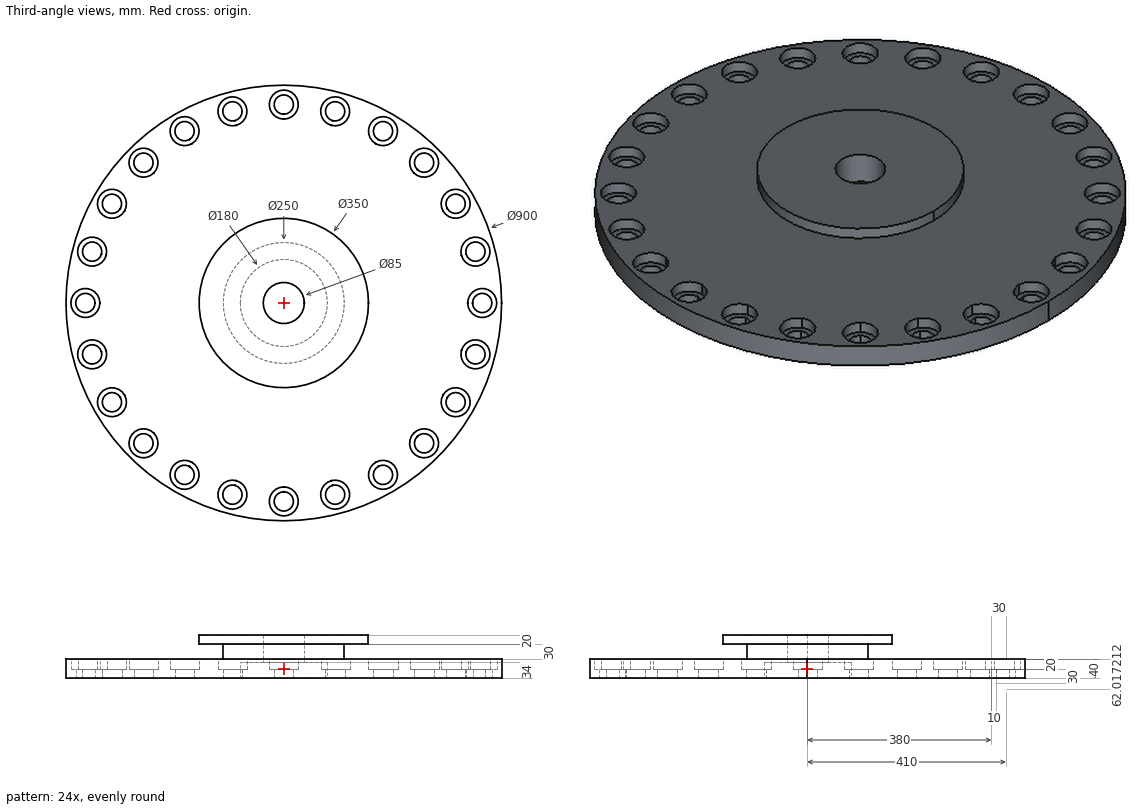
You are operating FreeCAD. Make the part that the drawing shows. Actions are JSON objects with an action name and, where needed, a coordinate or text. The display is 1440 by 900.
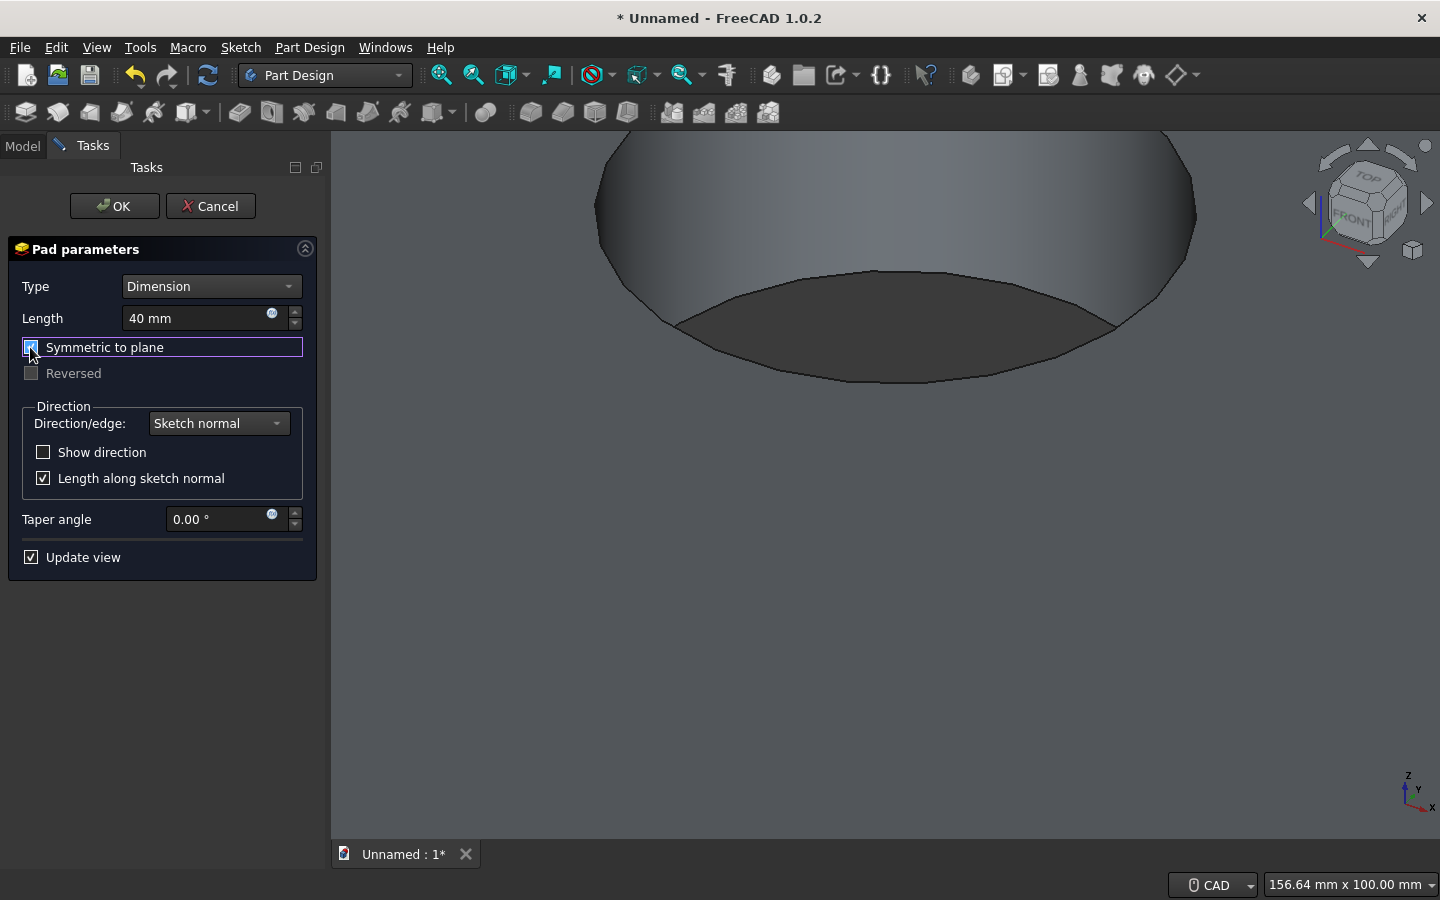
{"action": "left_click", "coordinate": [115, 206]}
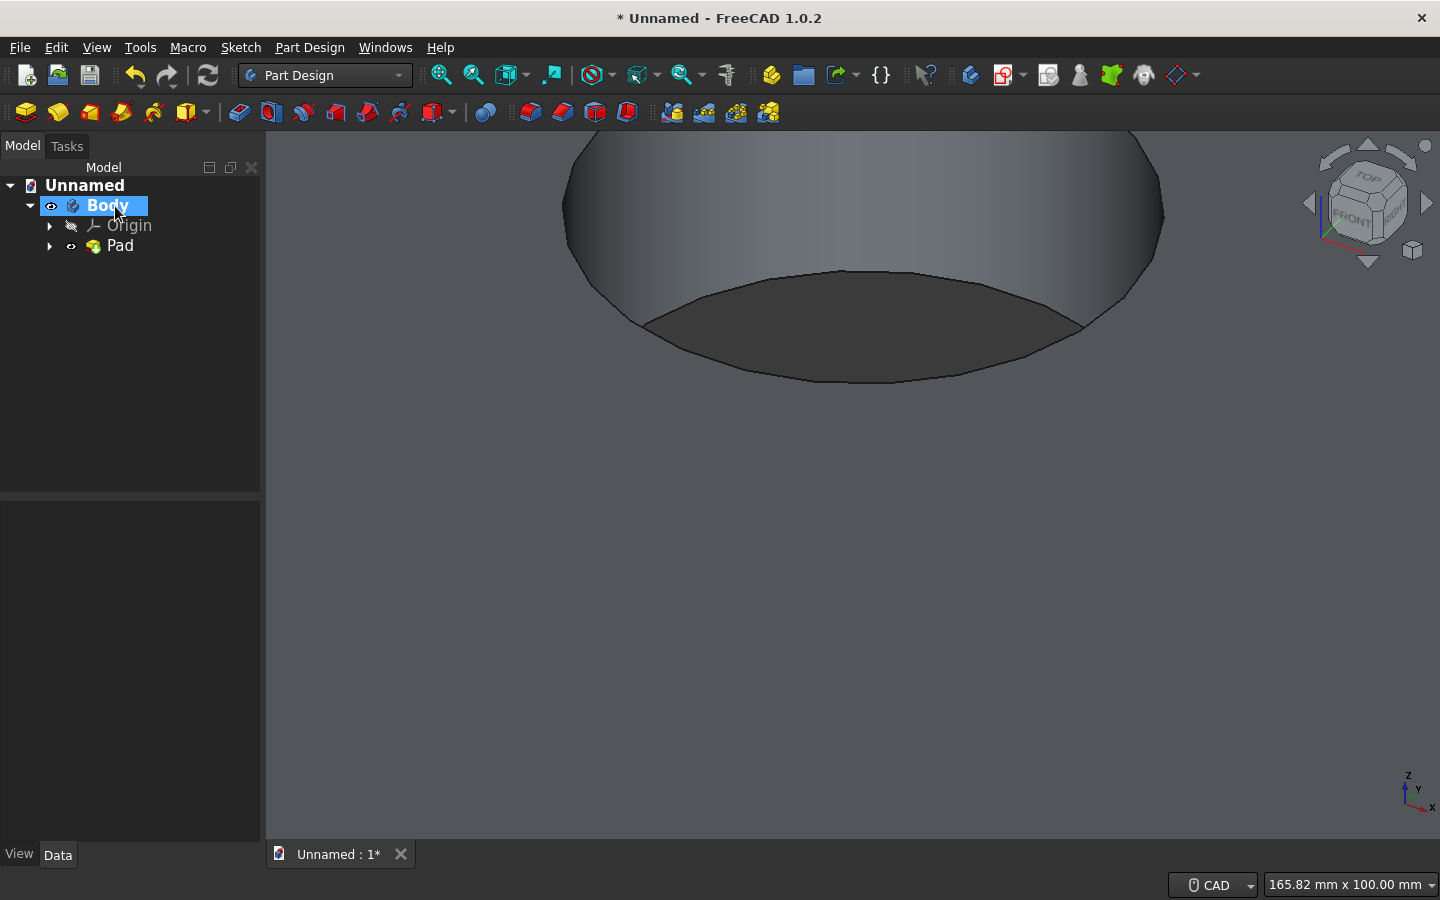
{"action": "key", "text": "v f"}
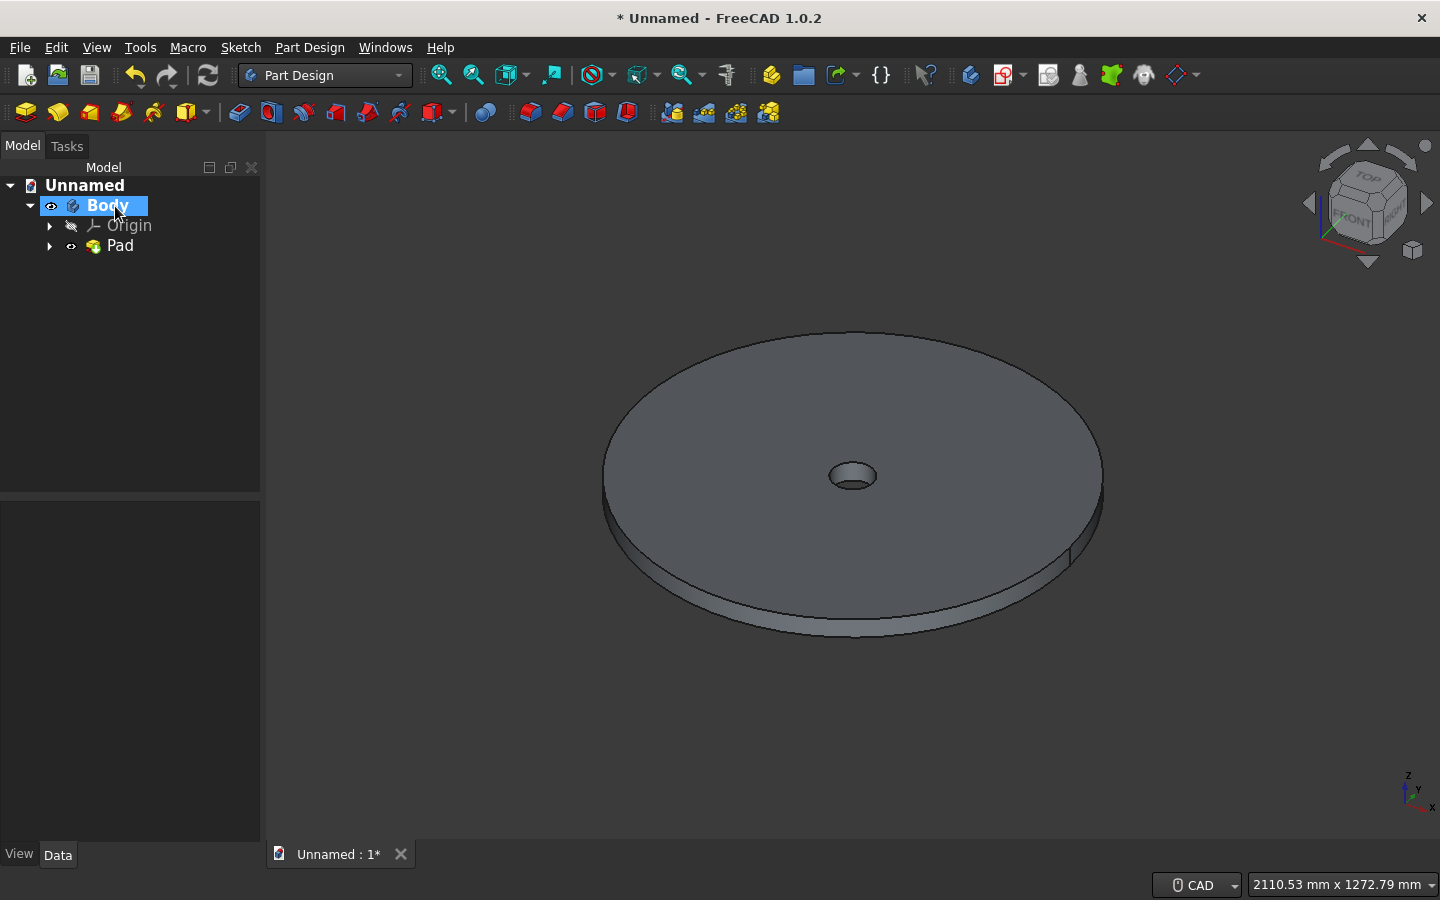
{"action": "left_click", "coordinate": [1004, 76]}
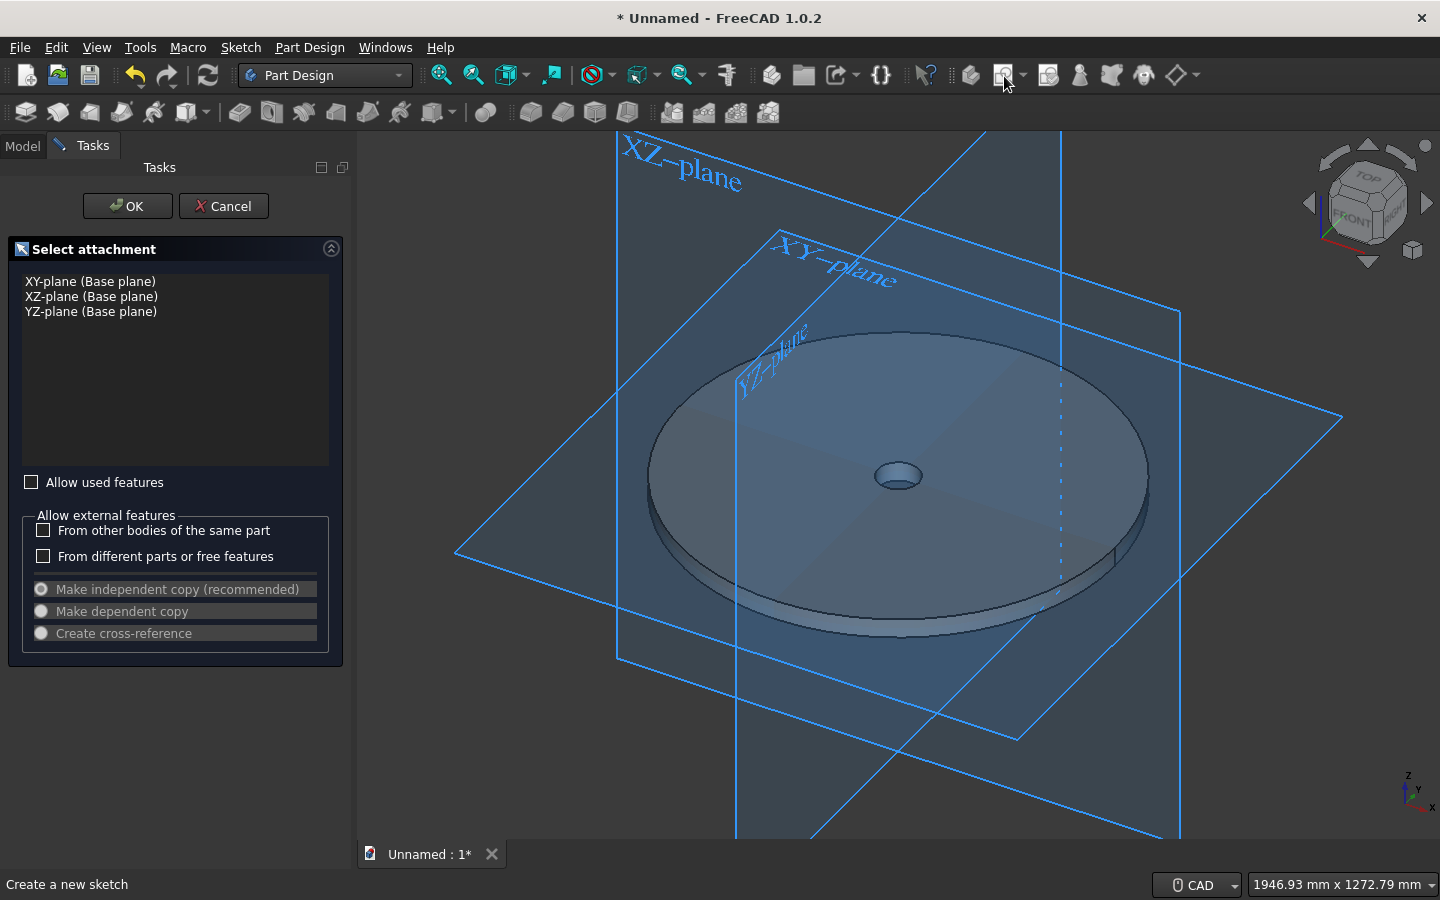
{"action": "left_click", "coordinate": [82, 312]}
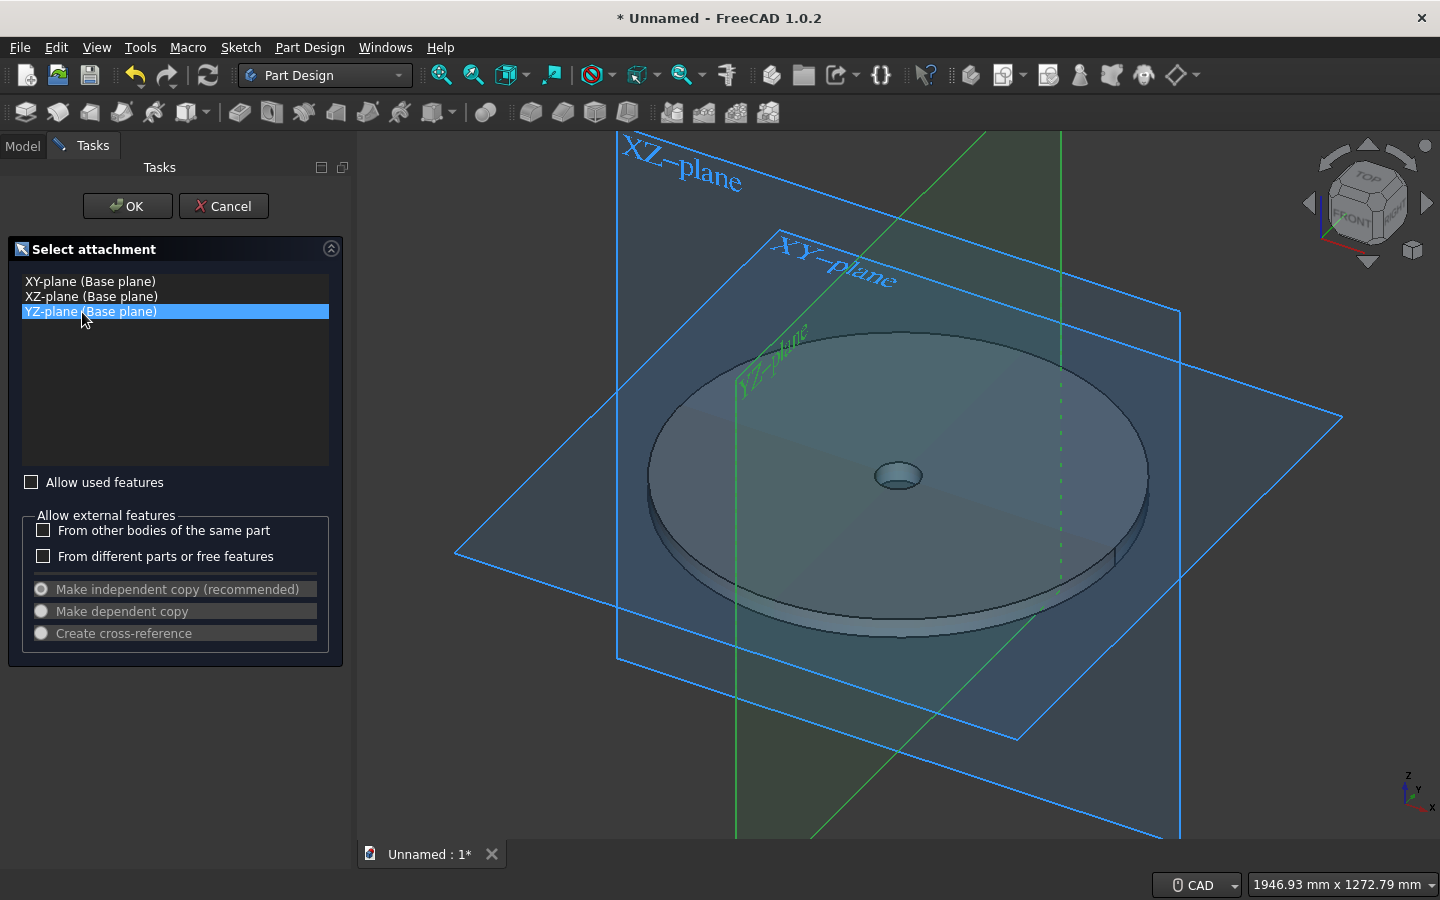
{"action": "left_click", "coordinate": [128, 206]}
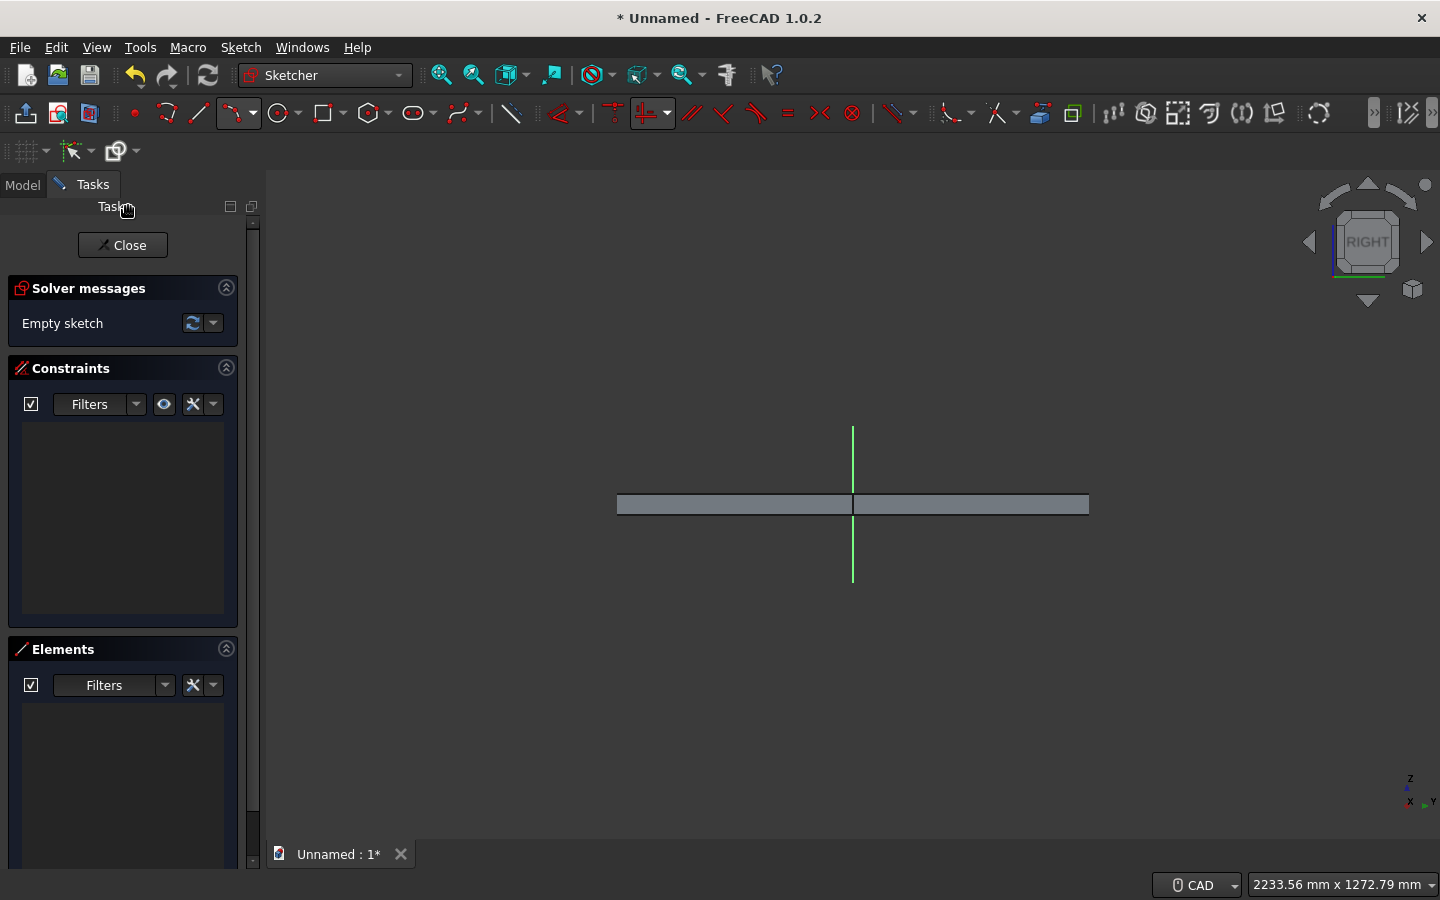
{"action": "left_click", "coordinate": [90, 114]}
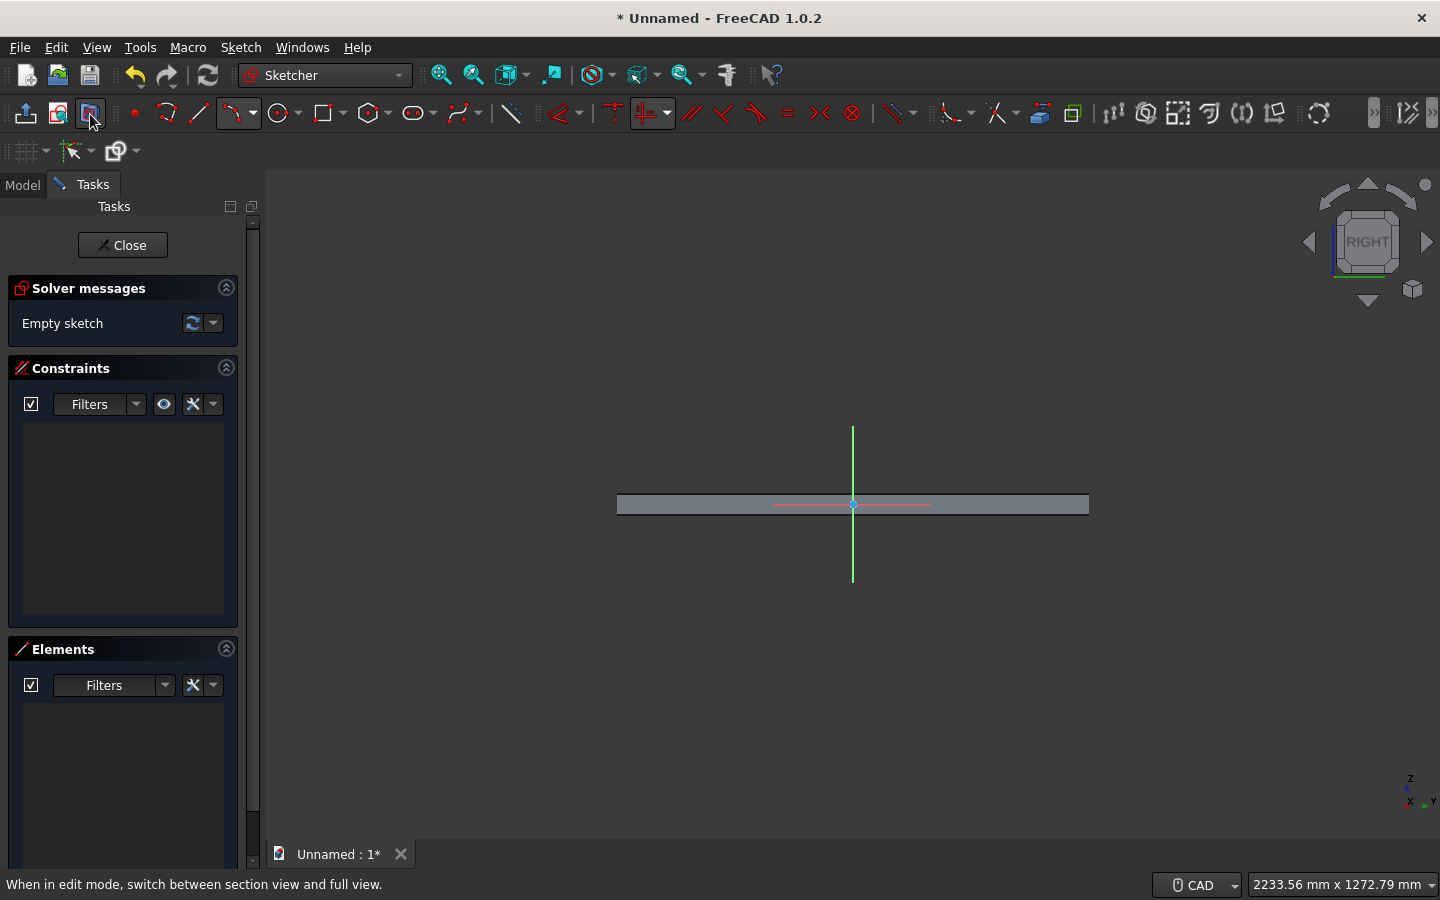
{"action": "scroll", "coordinate": [1095, 518], "scroll_direction": "up", "scroll_amount": 11}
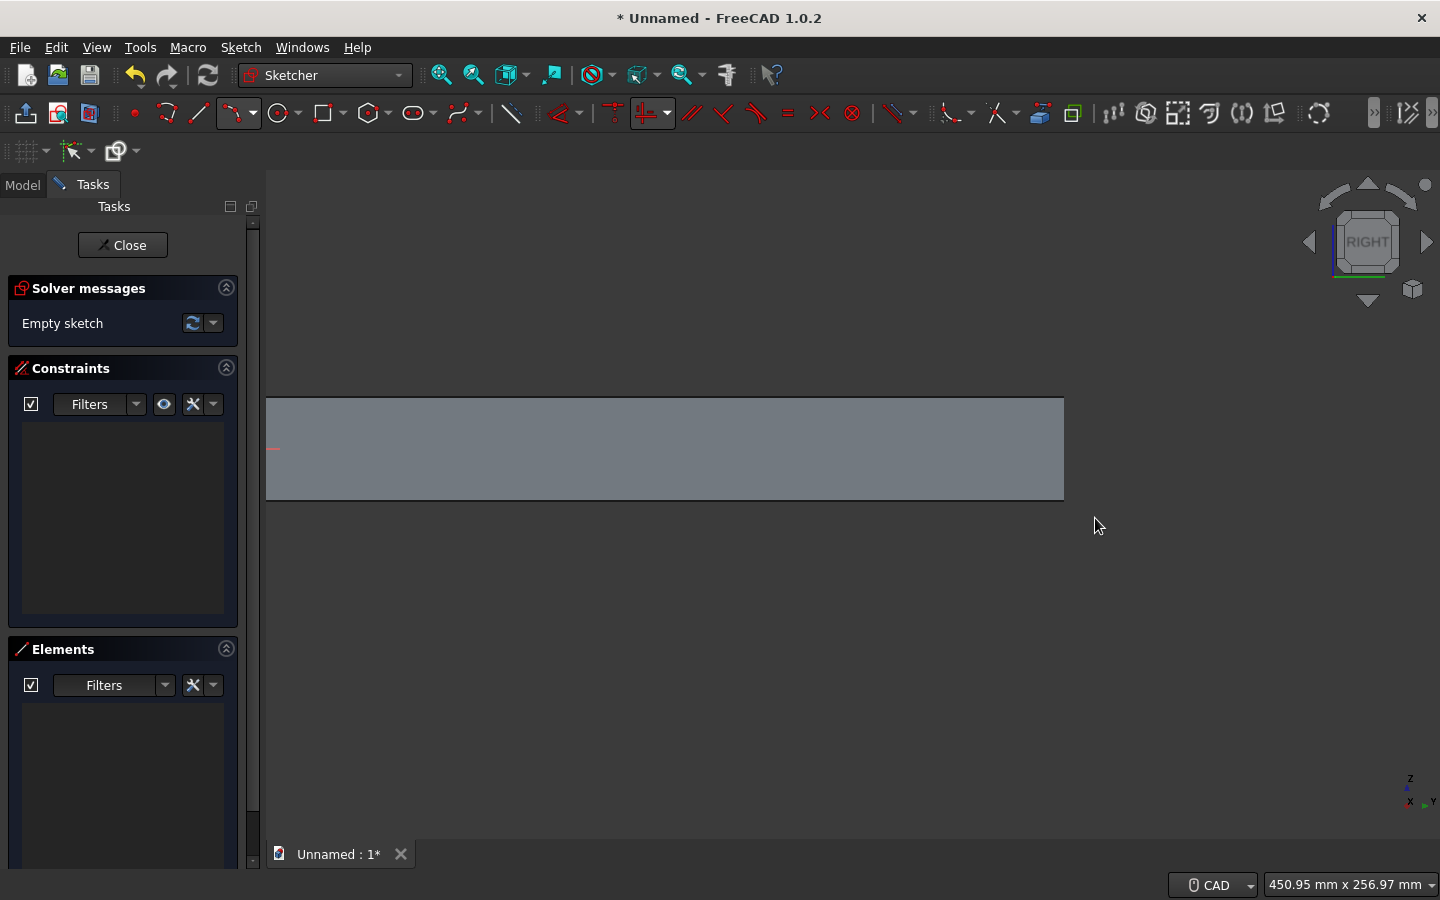
{"action": "key", "text": "g m"}